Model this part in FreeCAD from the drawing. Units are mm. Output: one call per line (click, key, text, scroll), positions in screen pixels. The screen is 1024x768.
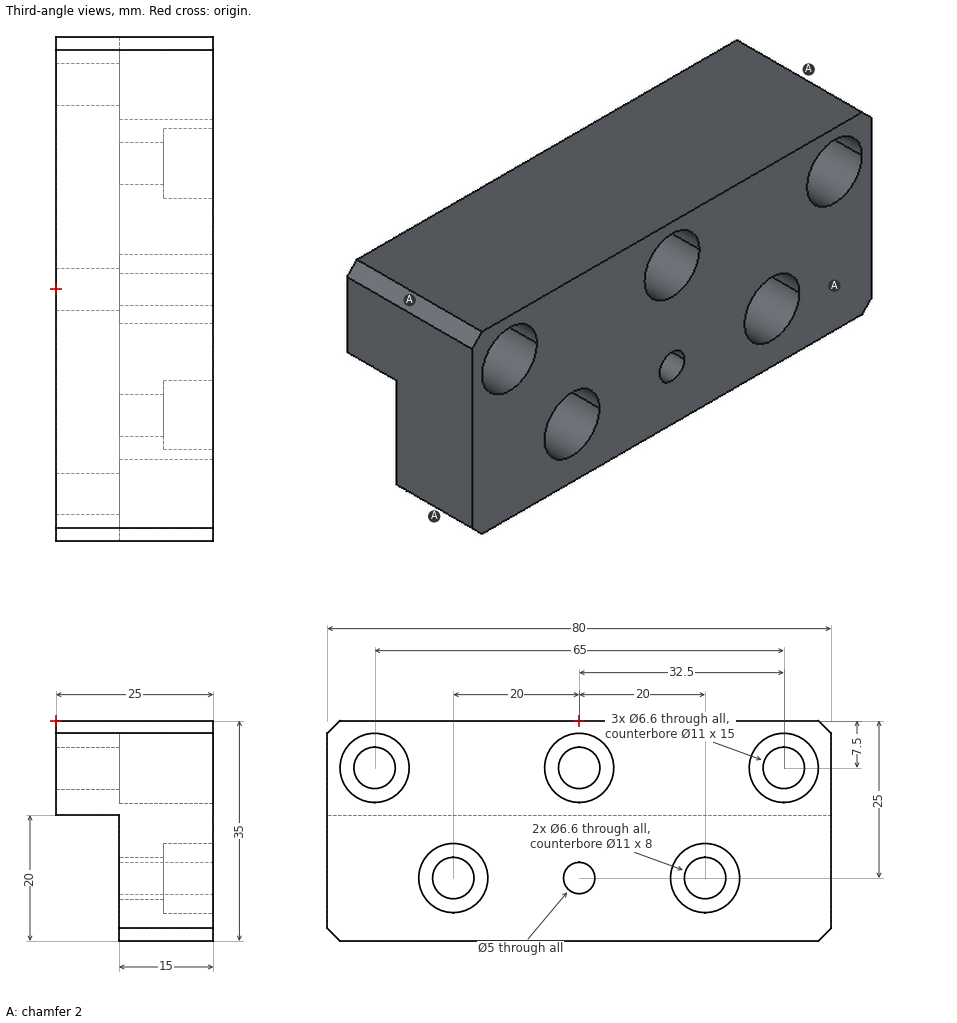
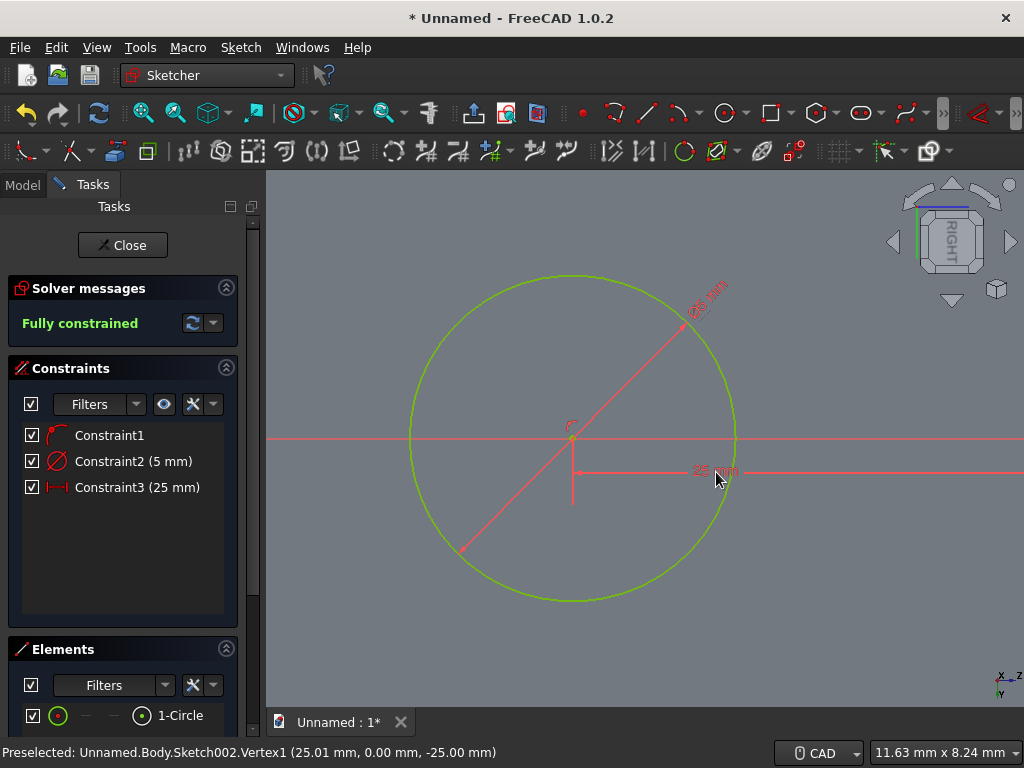
click(123, 245)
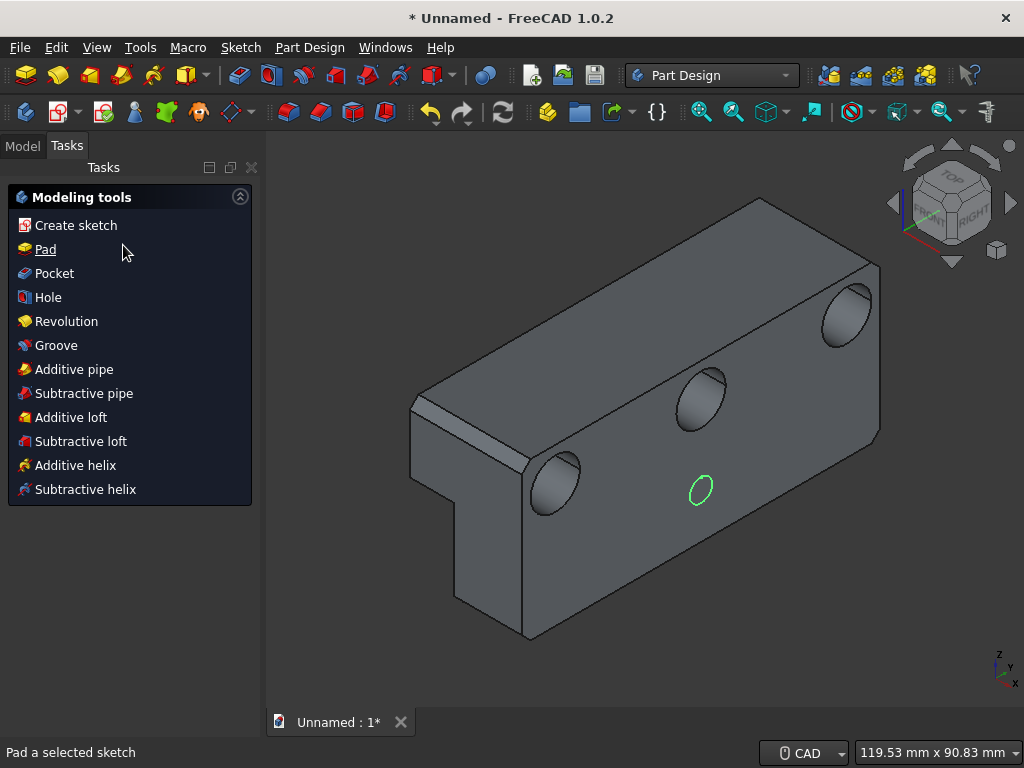
click(272, 76)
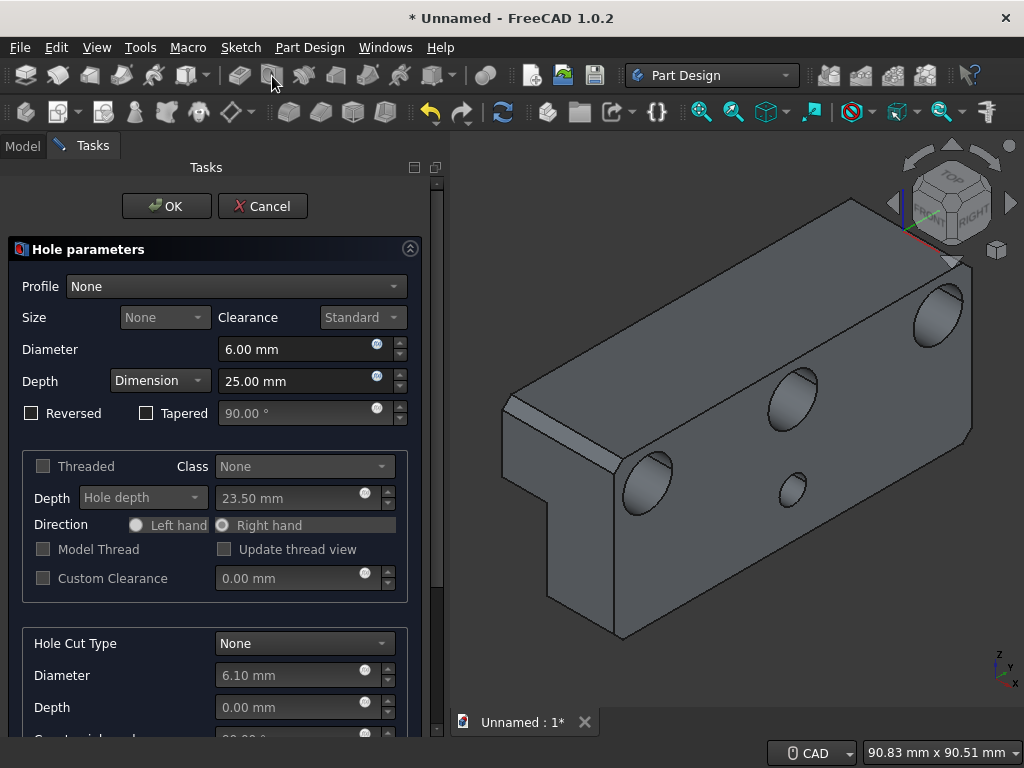
triple_click(305, 349)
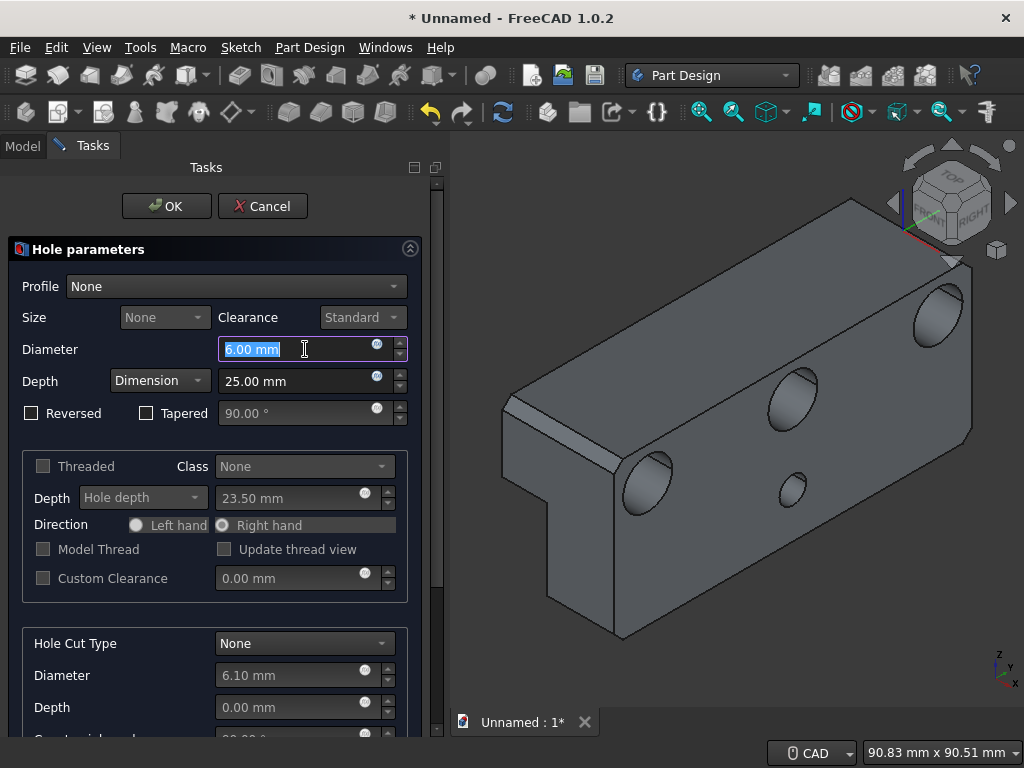
text(5)
key(Tab)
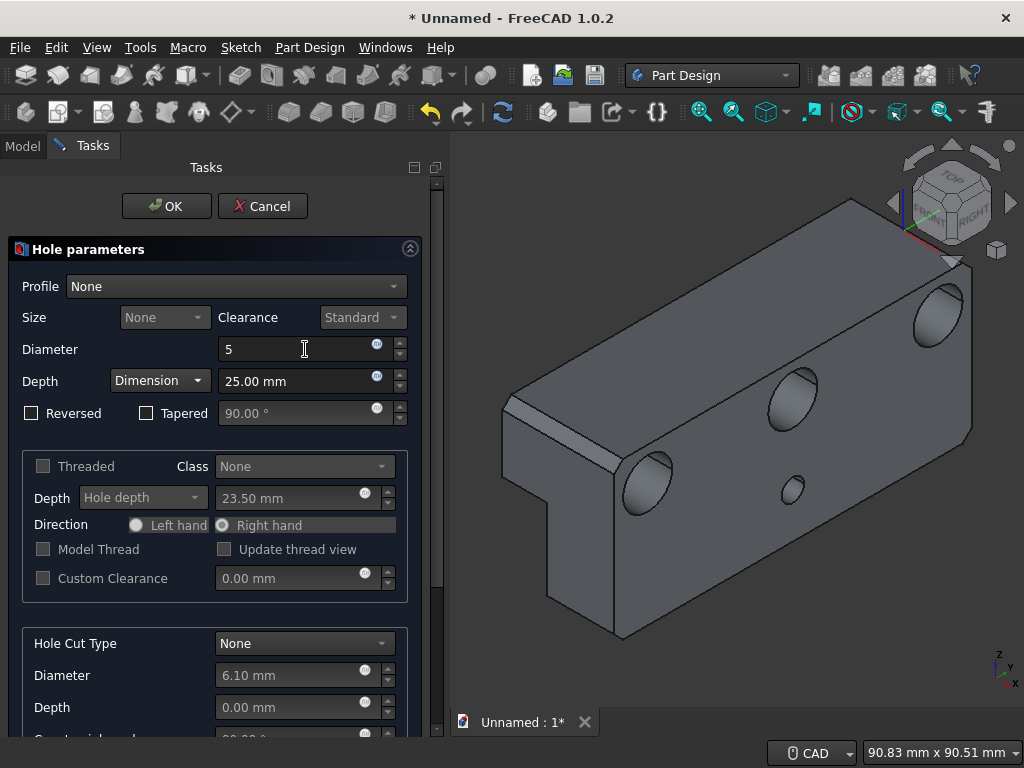
click(161, 380)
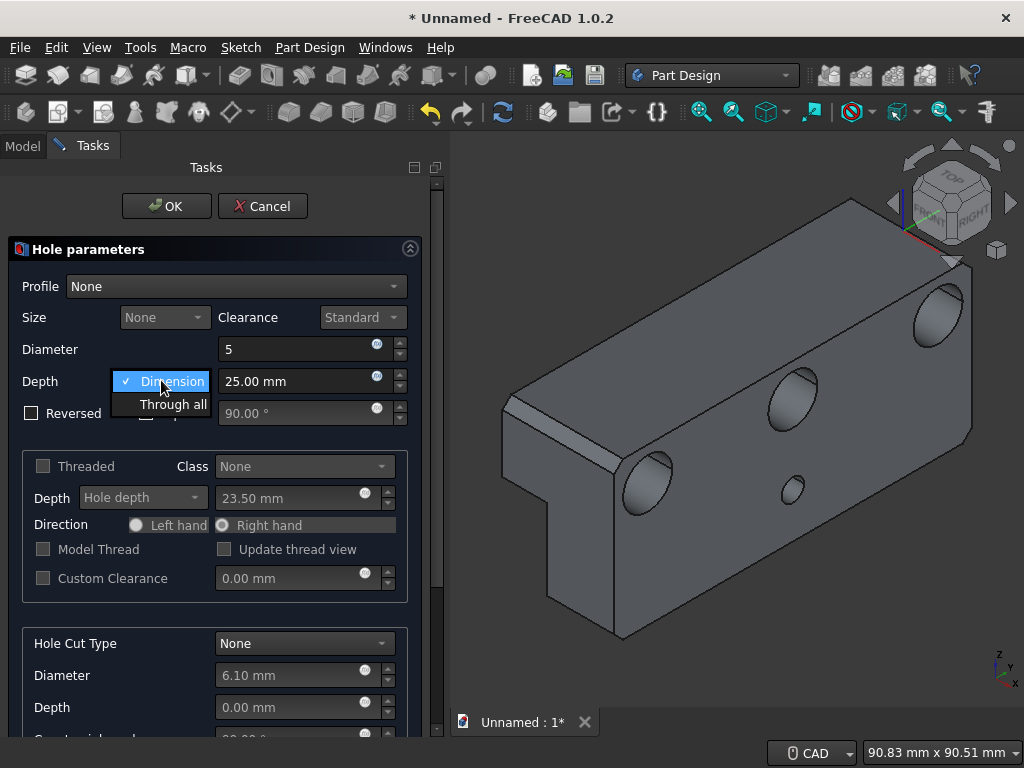
click(160, 404)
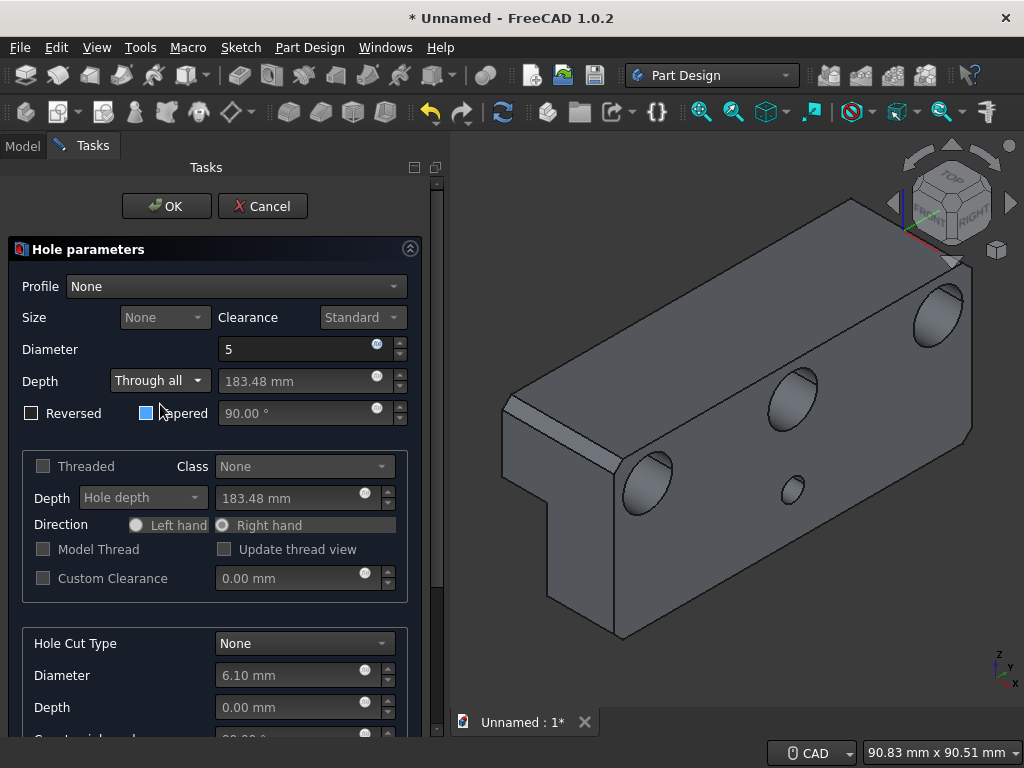
click(167, 206)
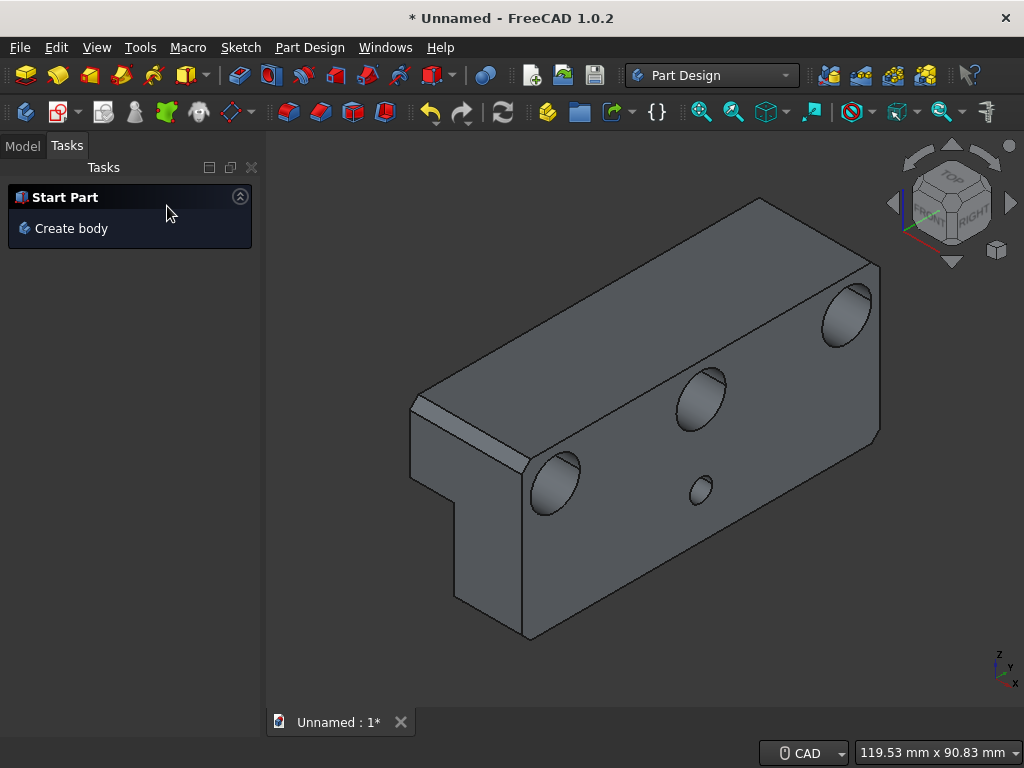
click(804, 417)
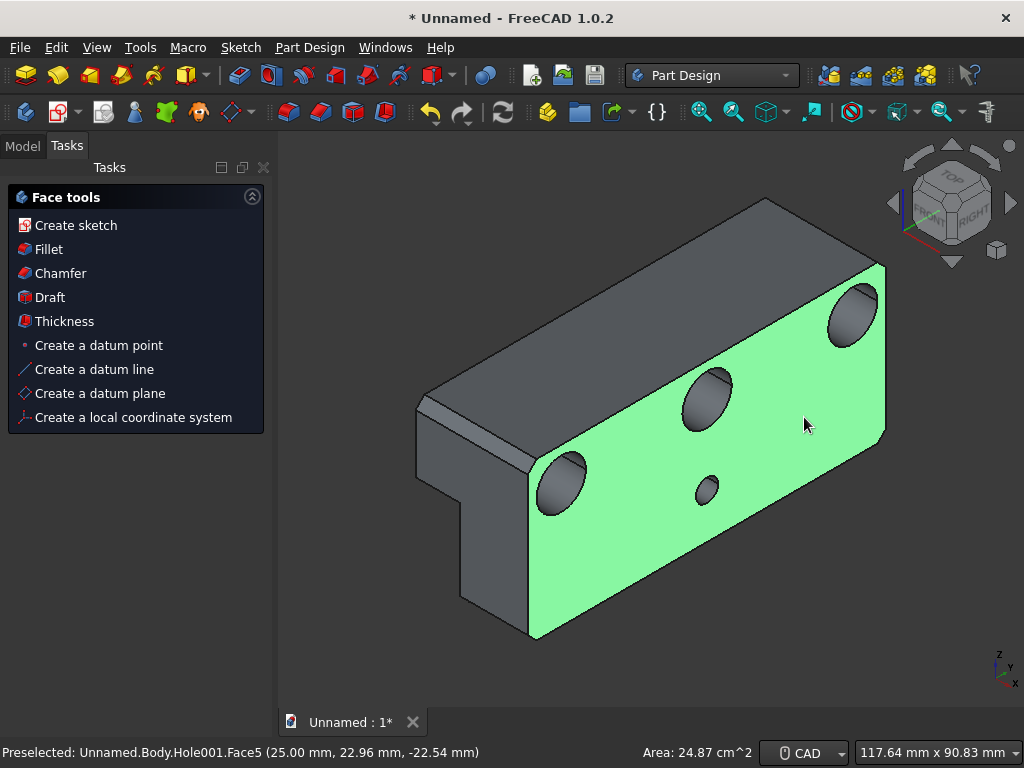
click(58, 112)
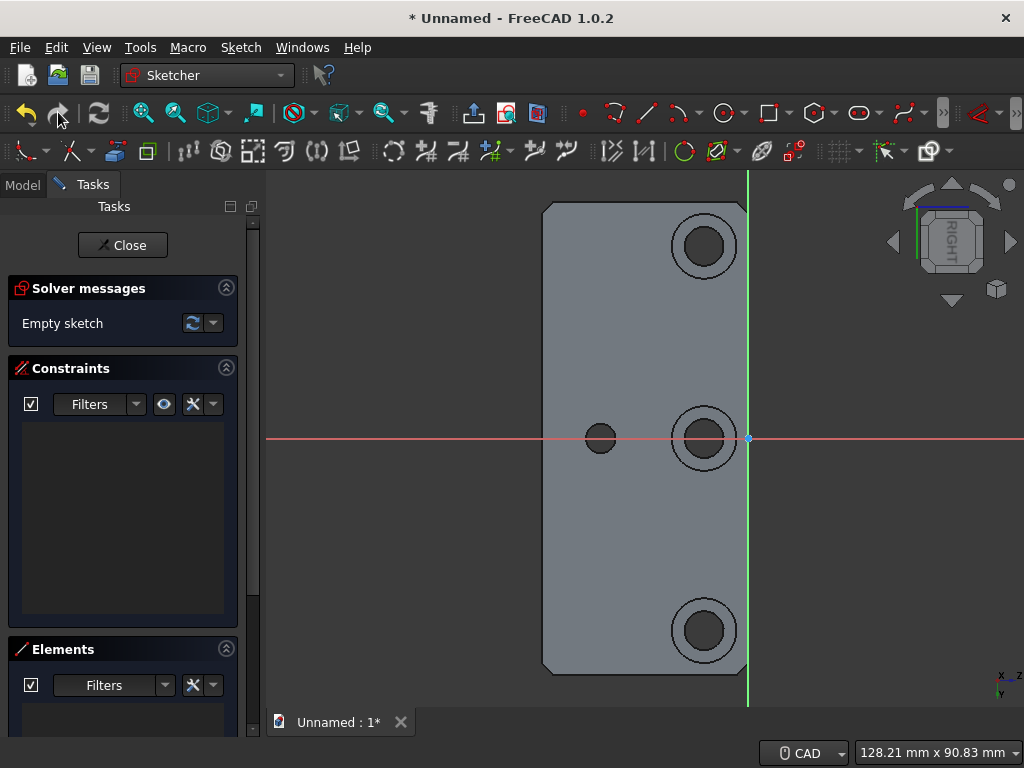
click(724, 114)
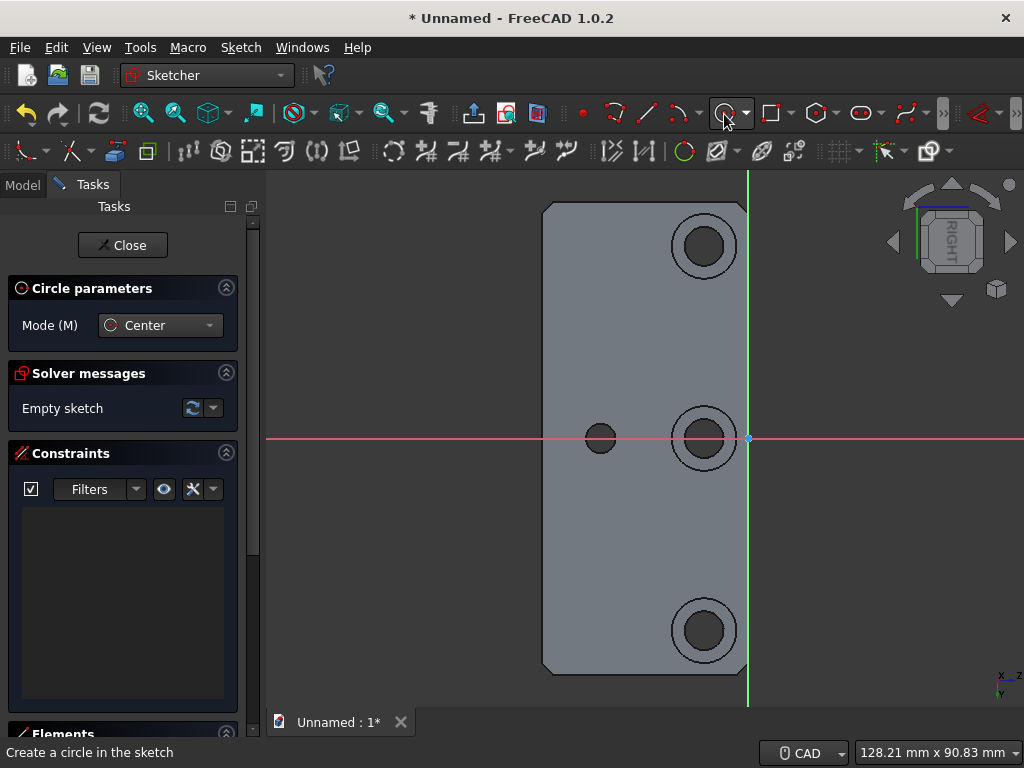
click(601, 557)
click(614, 543)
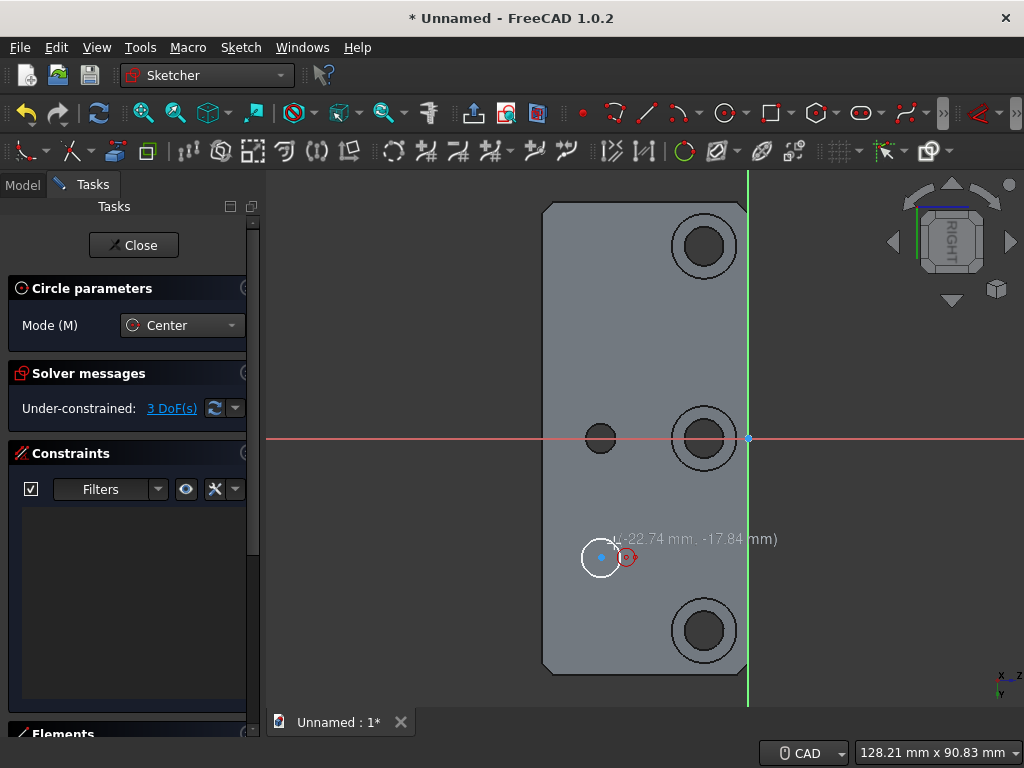
click(601, 320)
click(614, 306)
key(Escape)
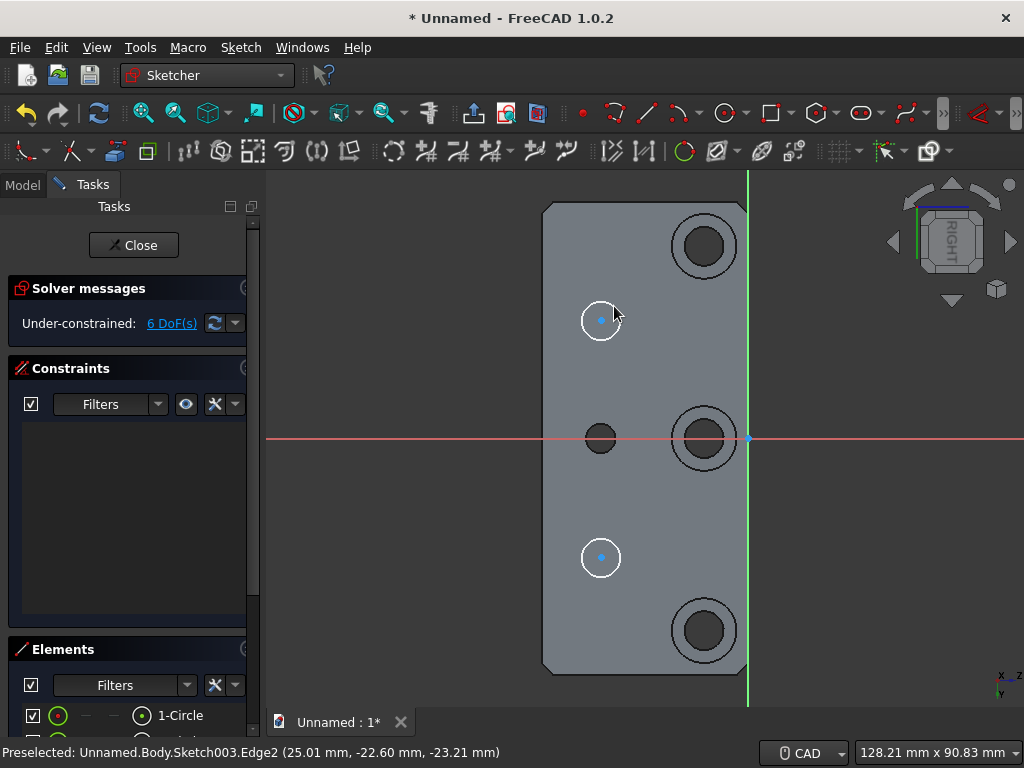
click(614, 544)